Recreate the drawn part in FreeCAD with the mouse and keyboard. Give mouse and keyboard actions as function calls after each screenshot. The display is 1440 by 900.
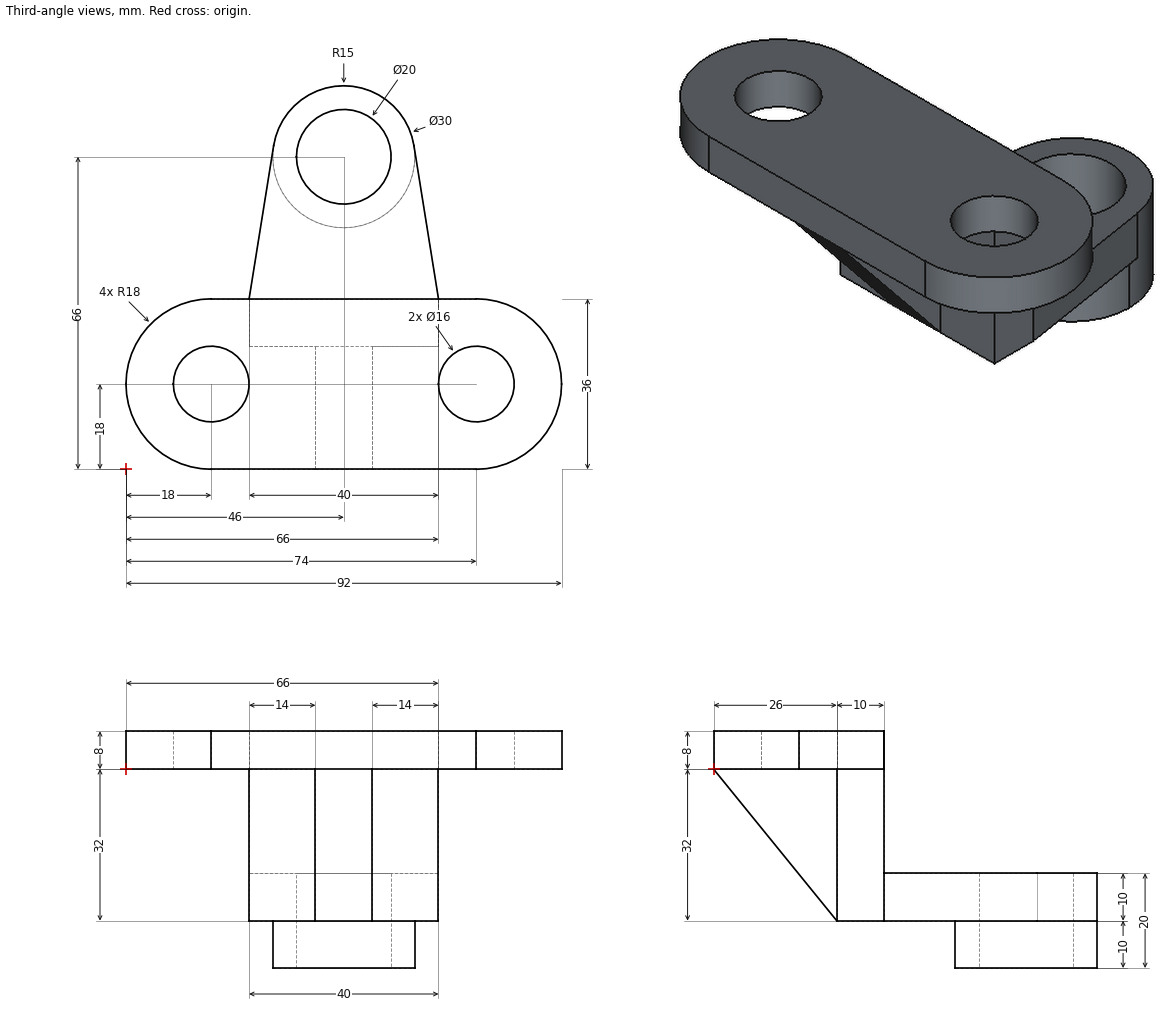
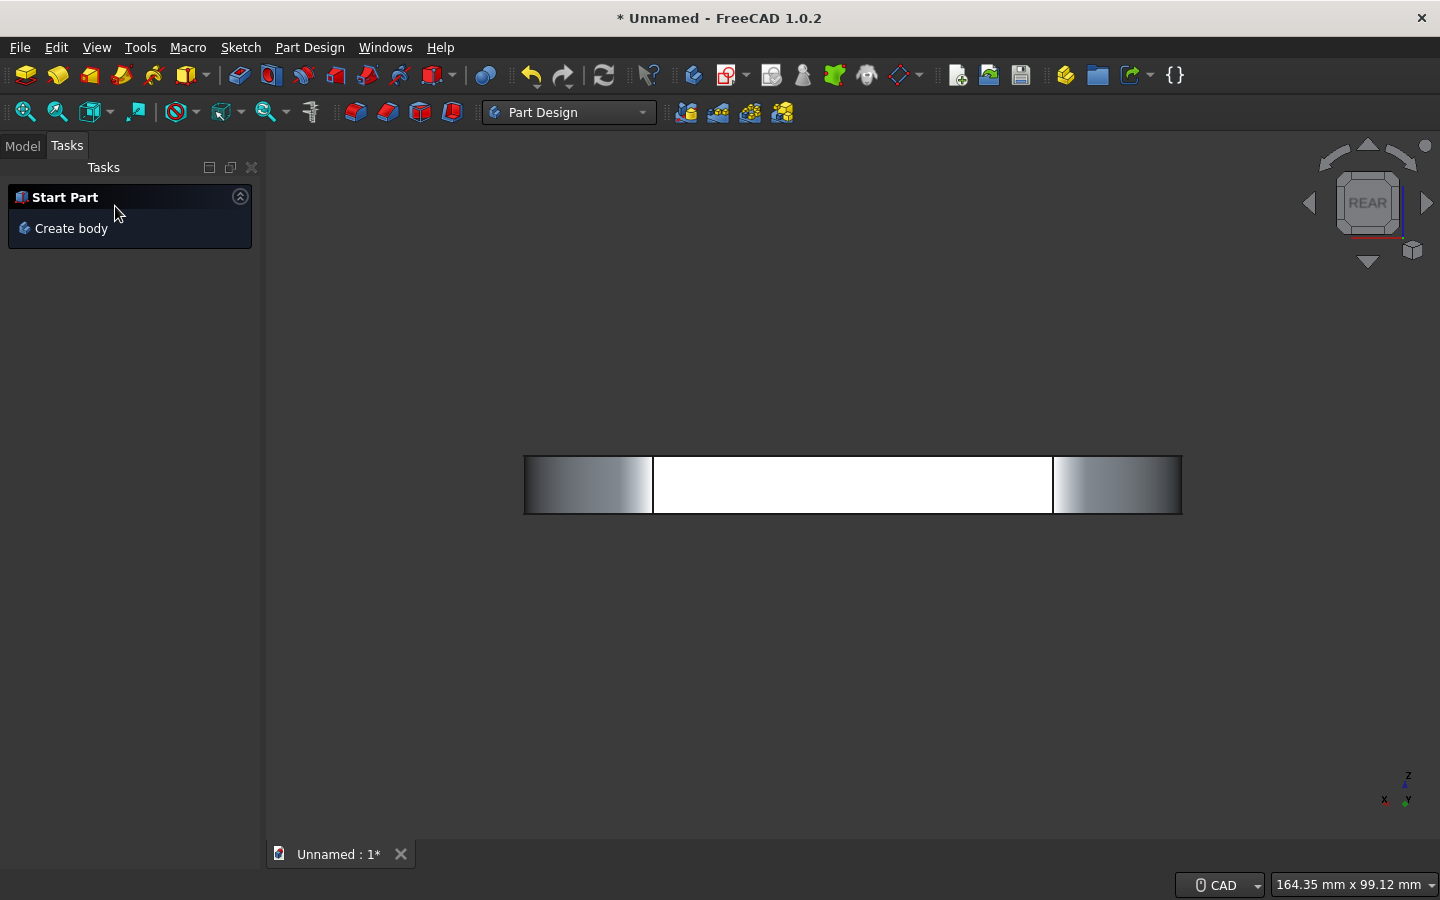
click(682, 484)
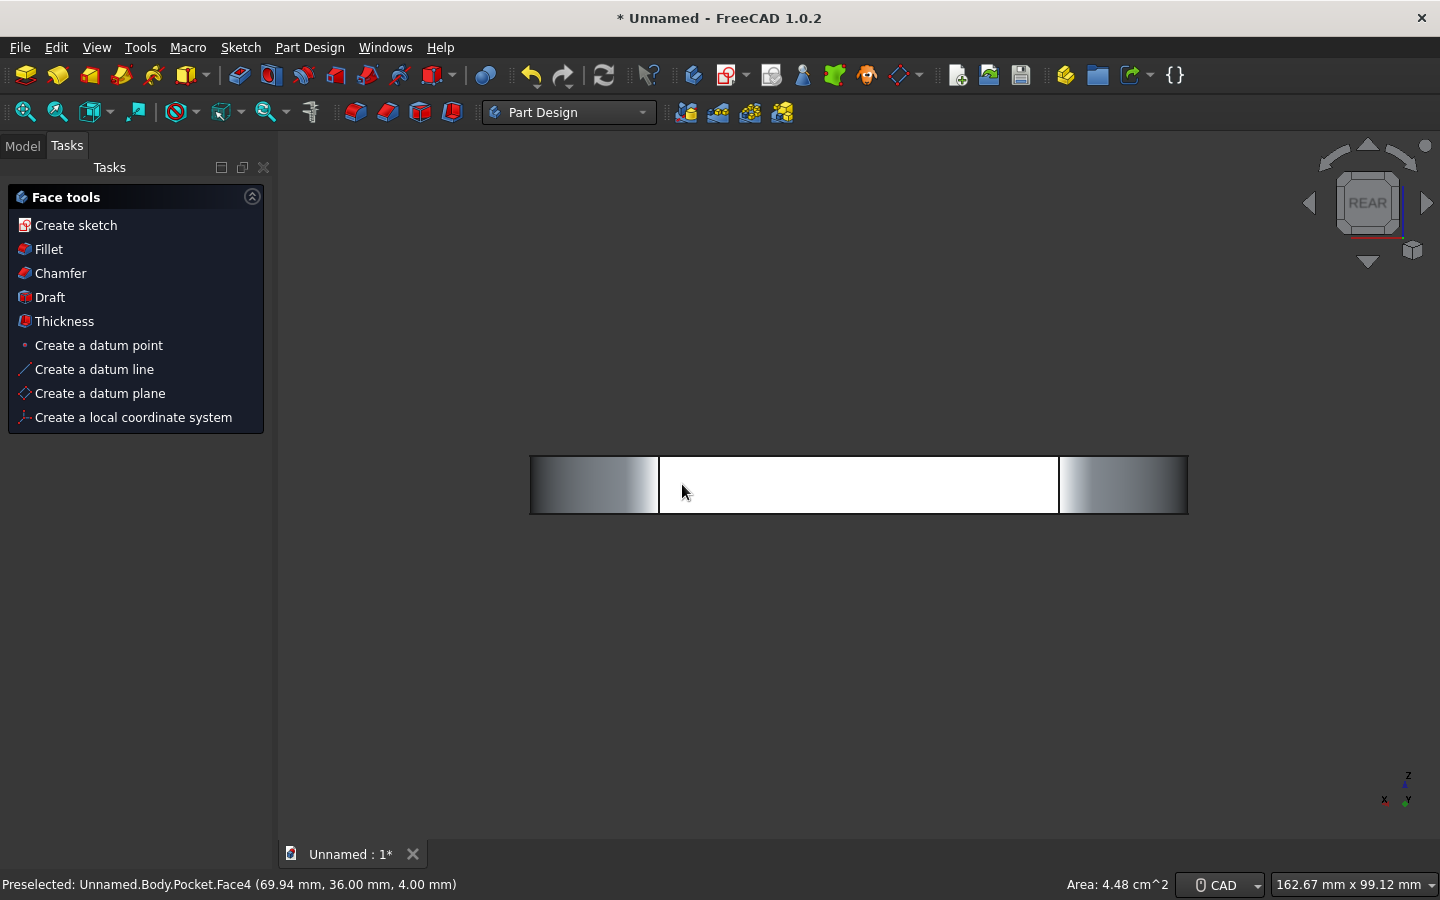
click(726, 76)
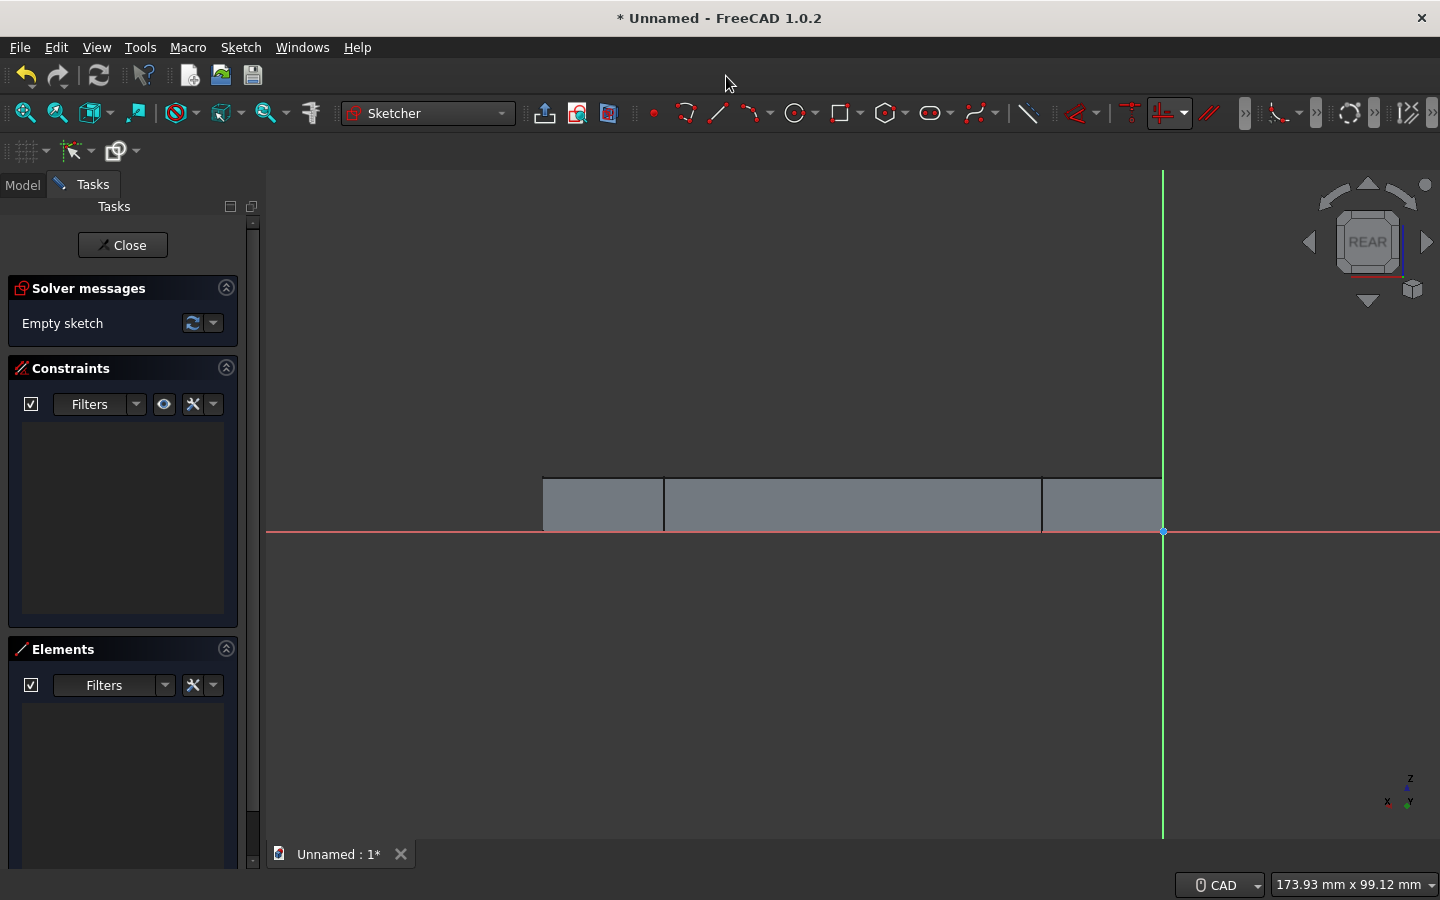
scroll(1258, 811, up, 2)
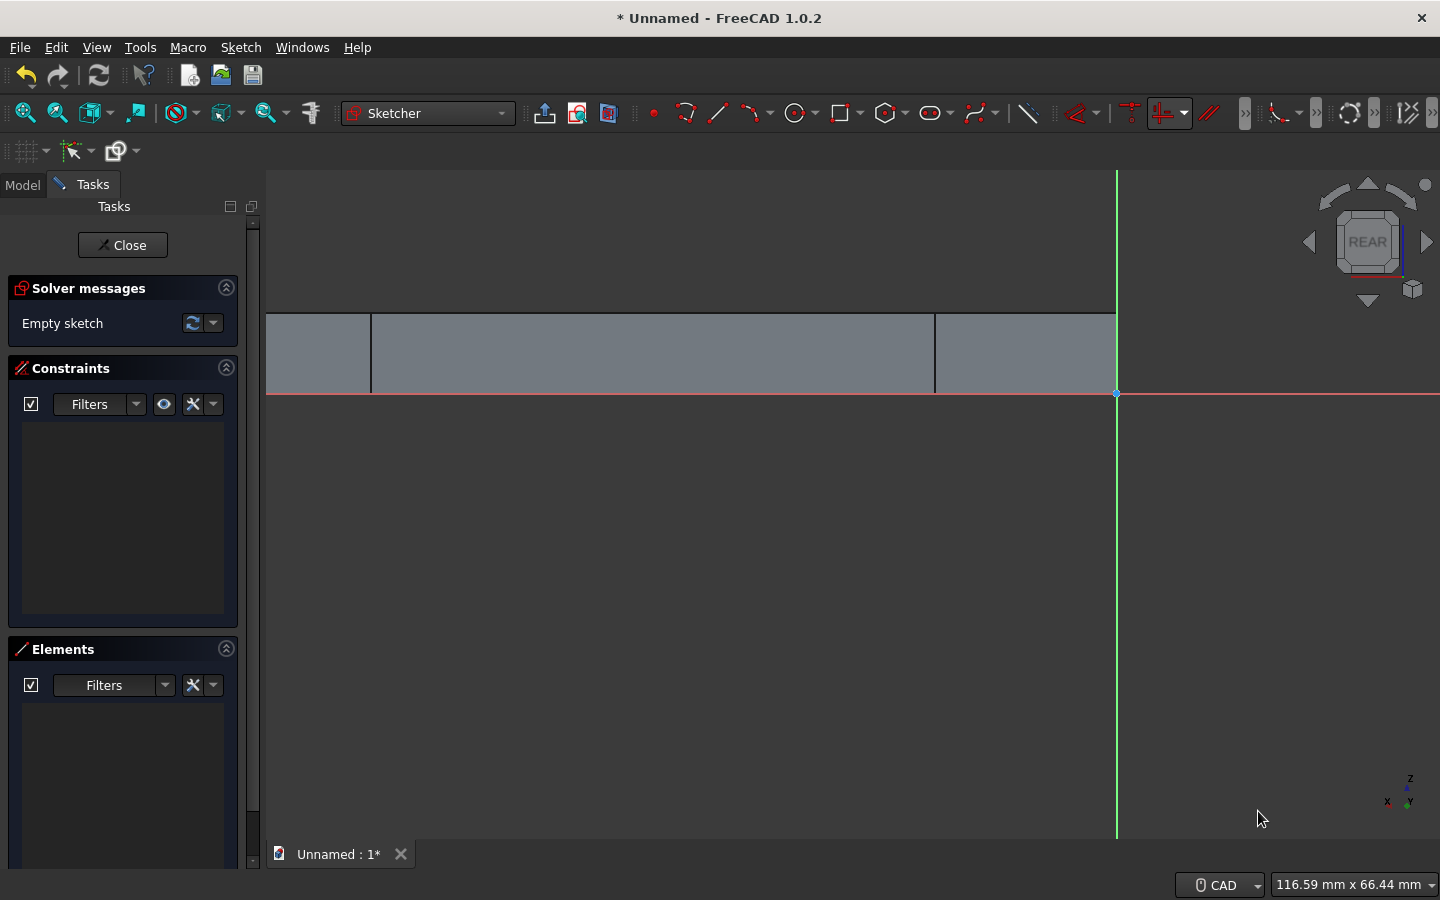
click(840, 114)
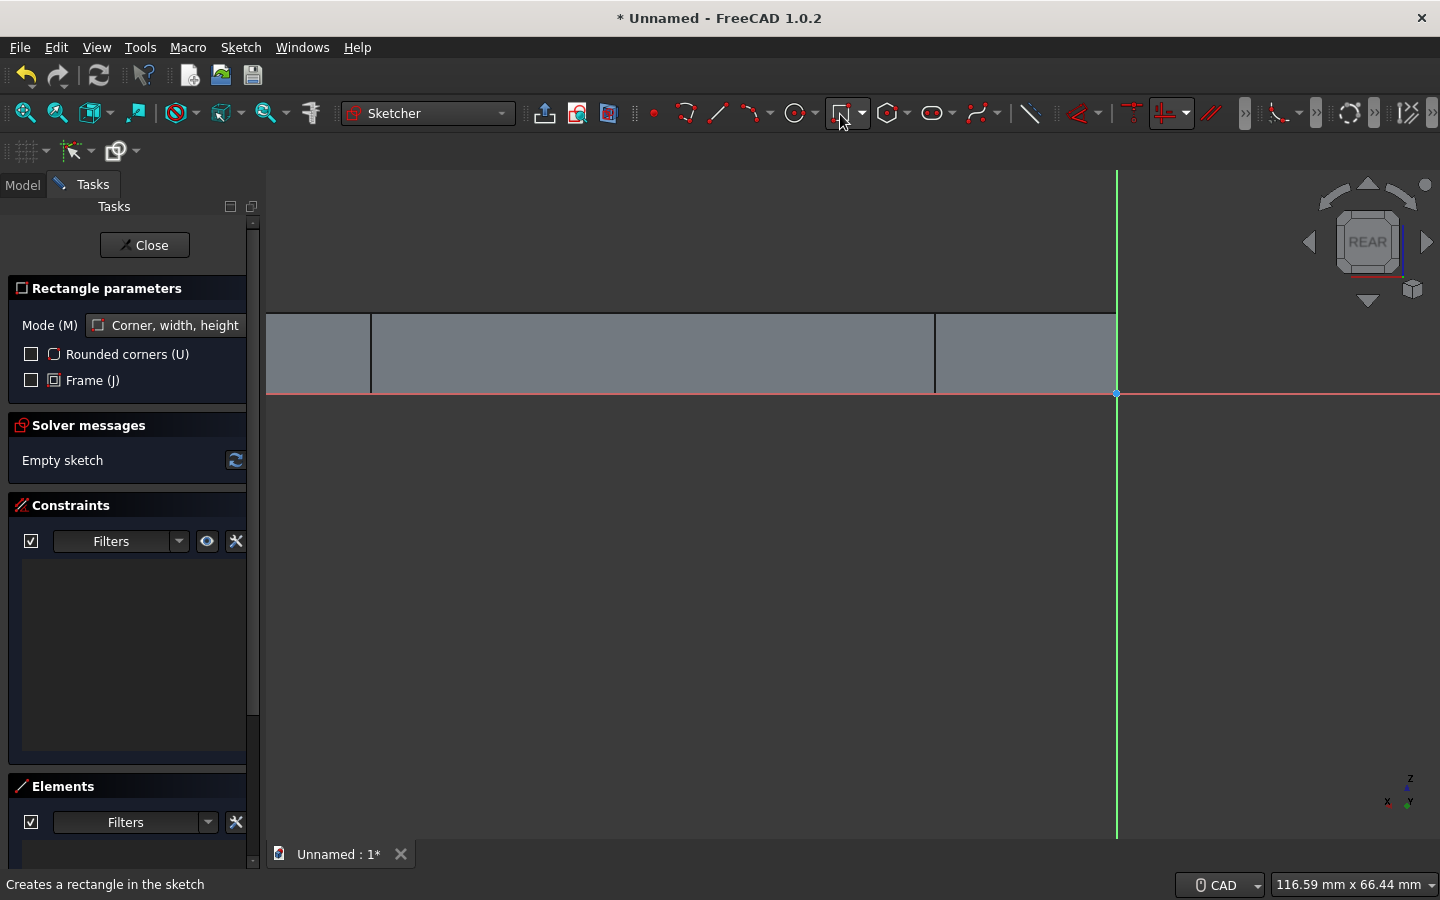
click(452, 394)
move(855, 716)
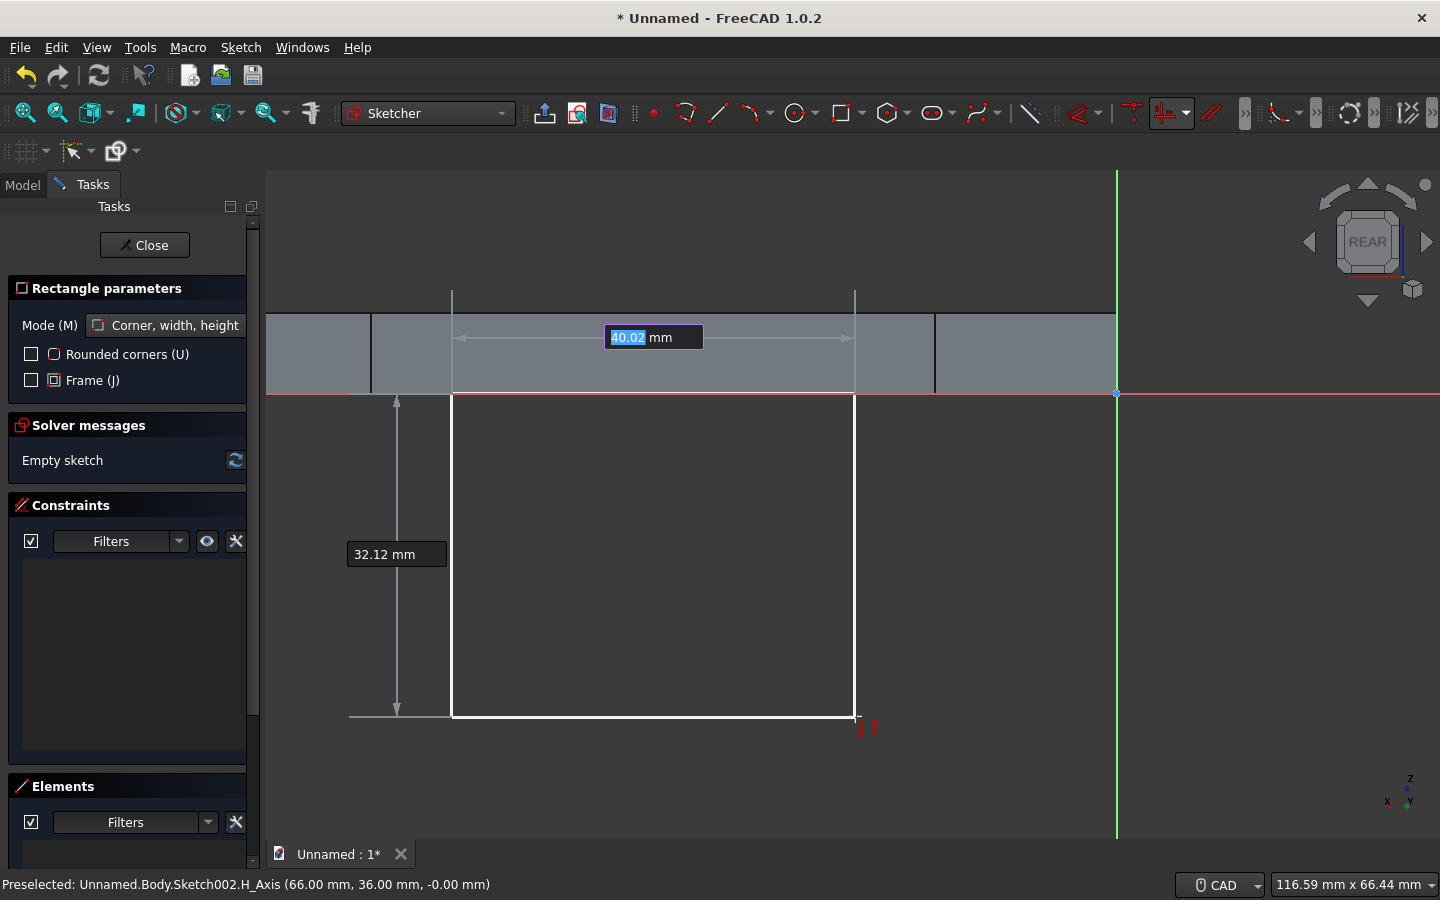
text(40)
key(Tab)
text(32)
key(Return)
key(Escape)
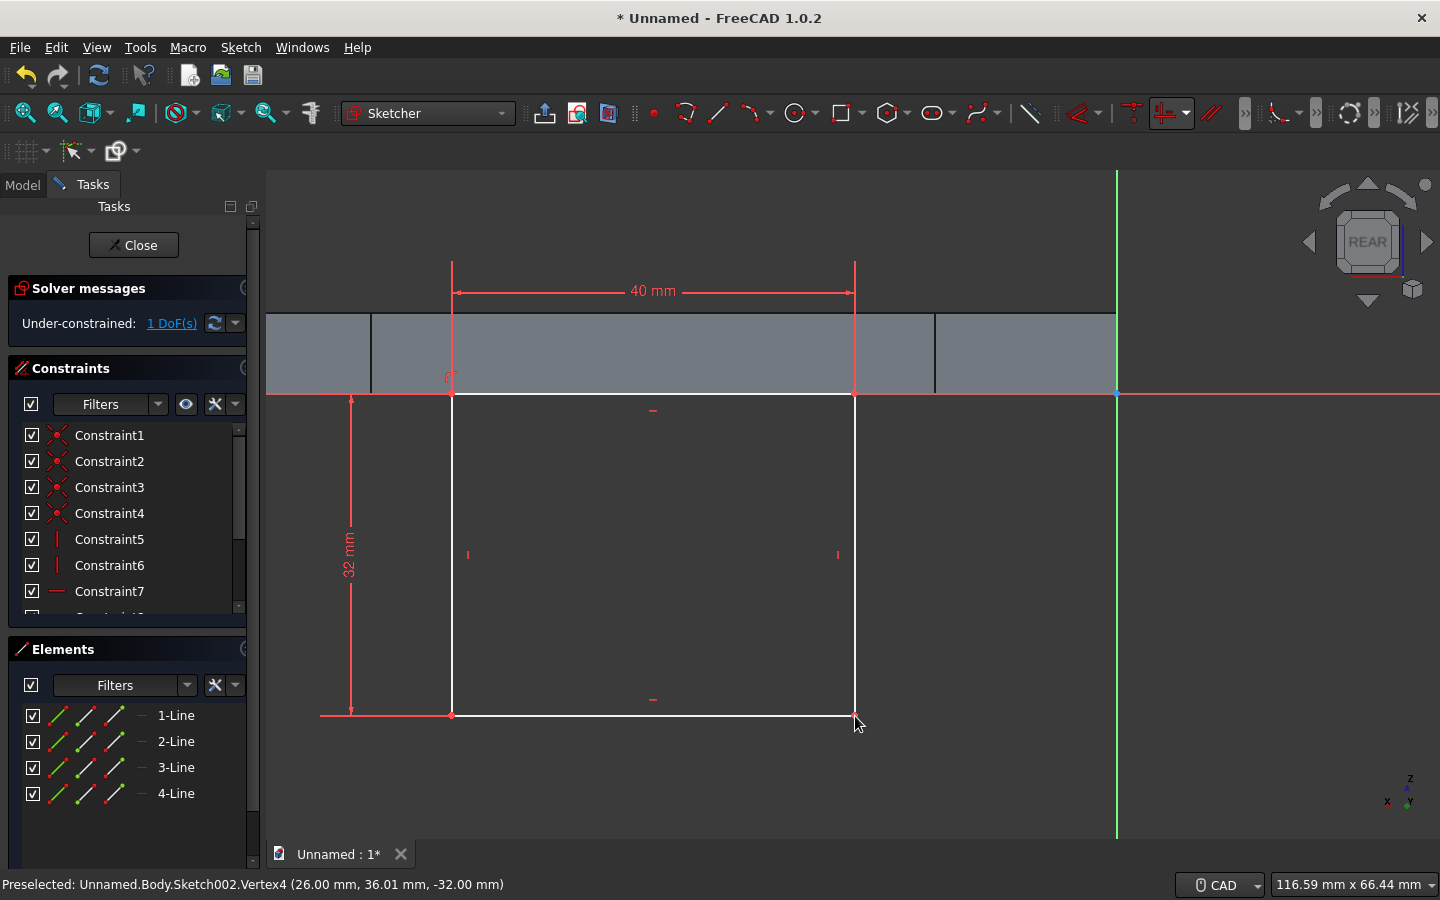
click(1078, 114)